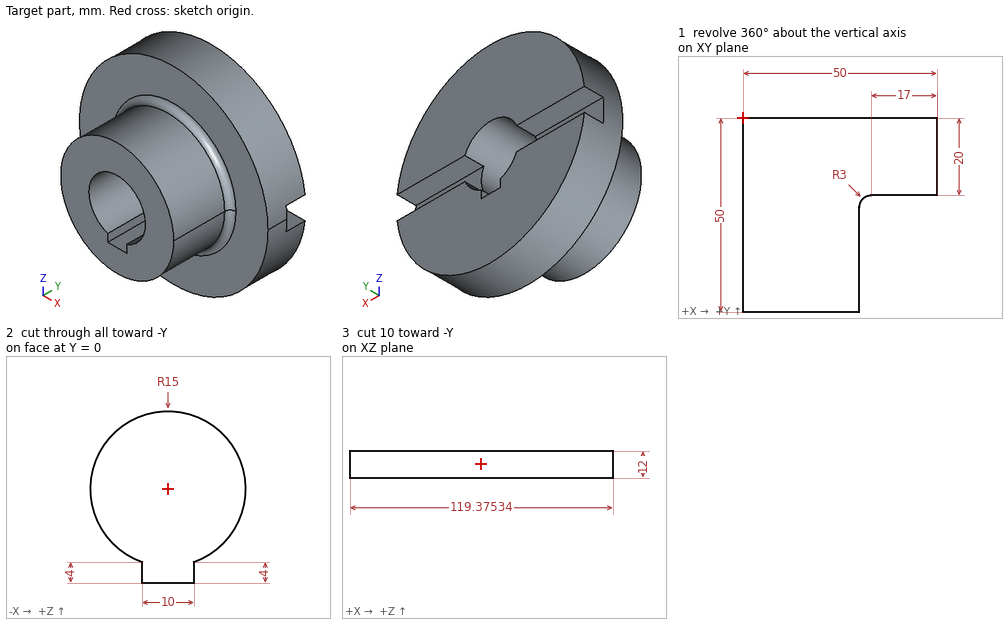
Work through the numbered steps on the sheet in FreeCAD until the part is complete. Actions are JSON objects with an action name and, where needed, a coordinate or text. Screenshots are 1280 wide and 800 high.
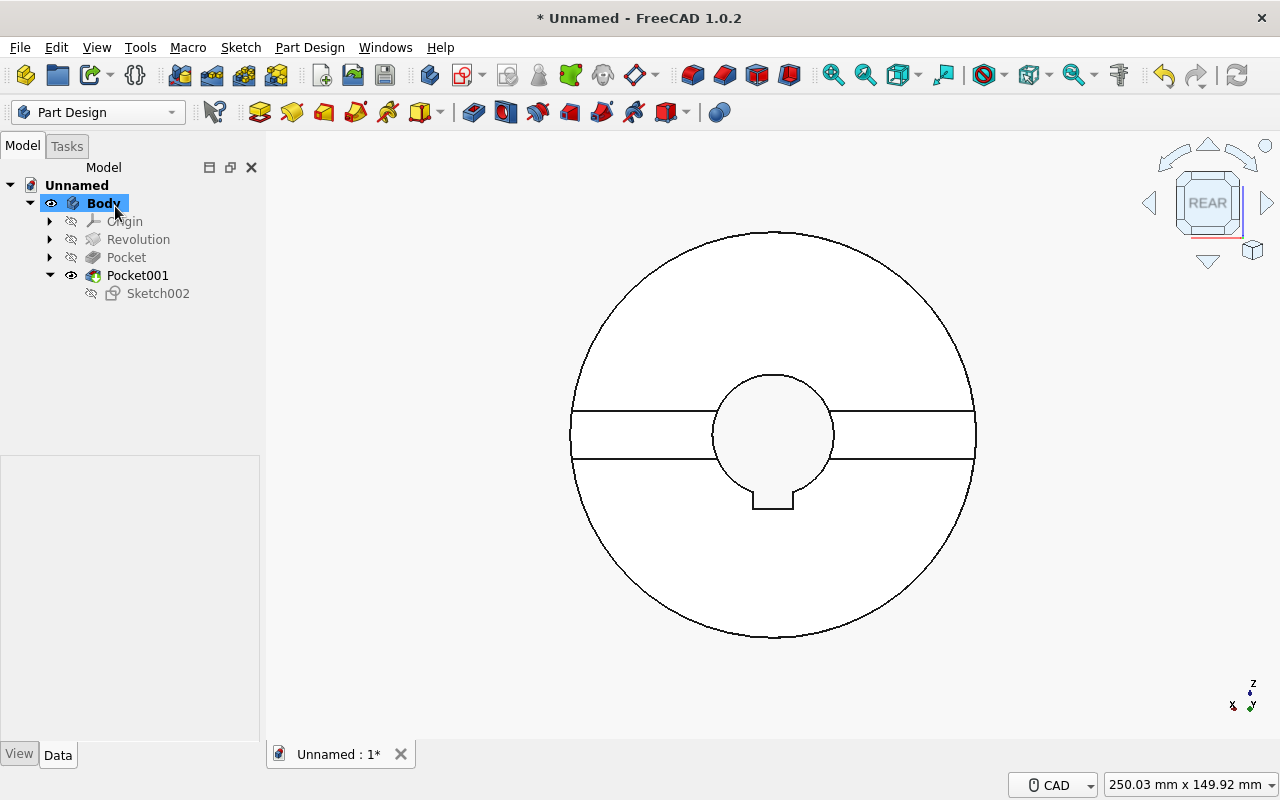
{"action": "key", "text": "0"}